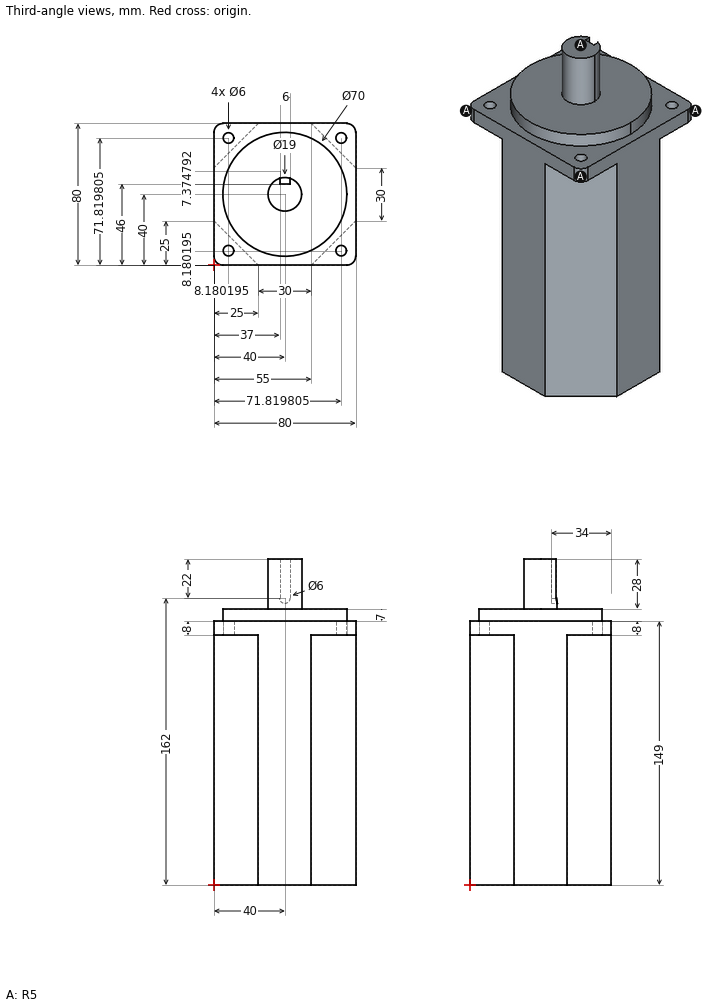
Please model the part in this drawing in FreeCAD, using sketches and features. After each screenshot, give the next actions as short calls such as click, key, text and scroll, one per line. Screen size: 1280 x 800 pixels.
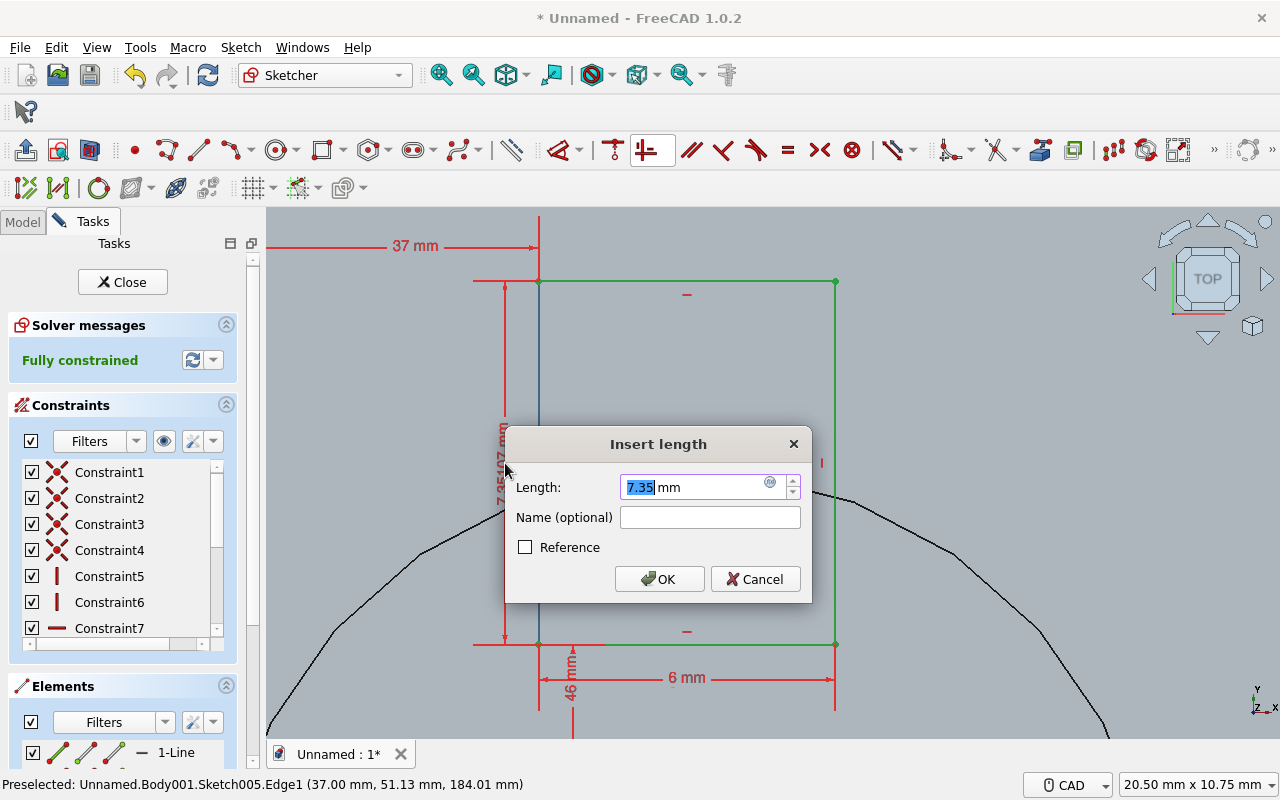
text(7.374792)
key(Return)
key(Escape)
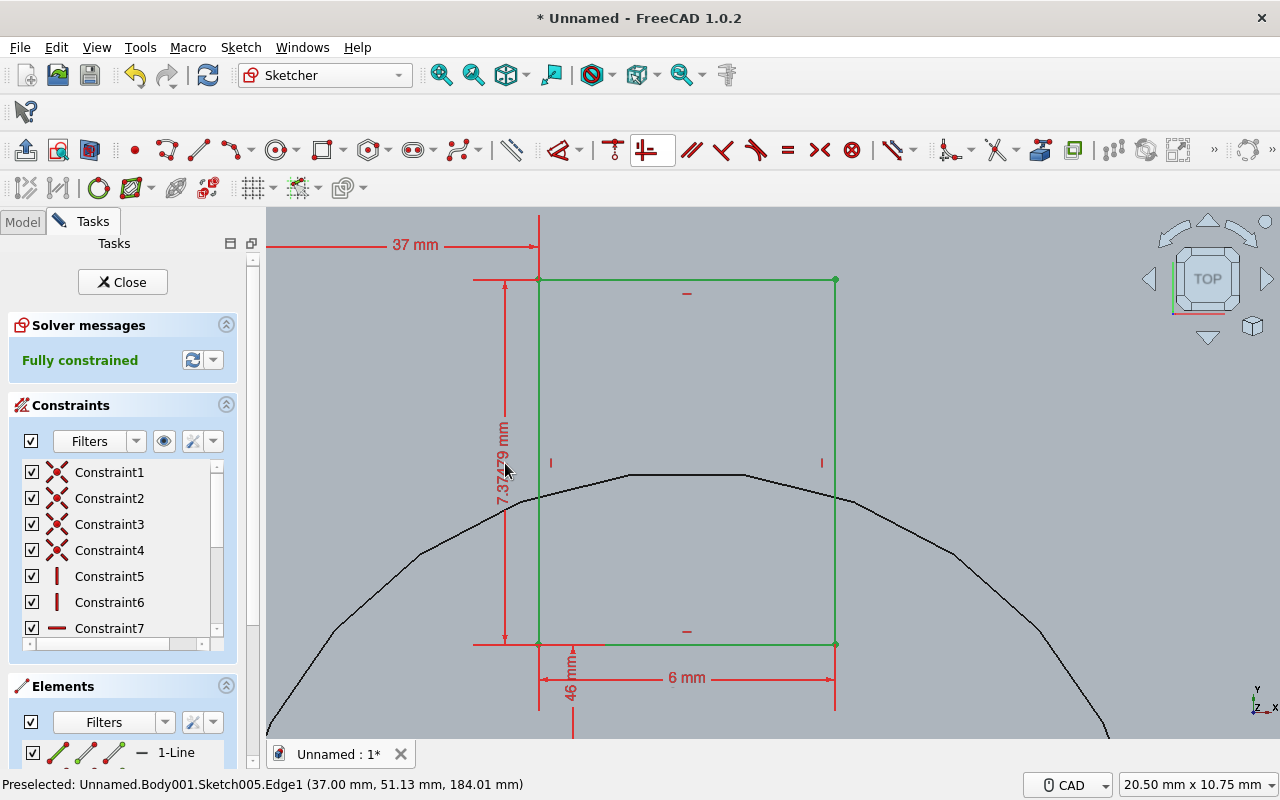
click(123, 282)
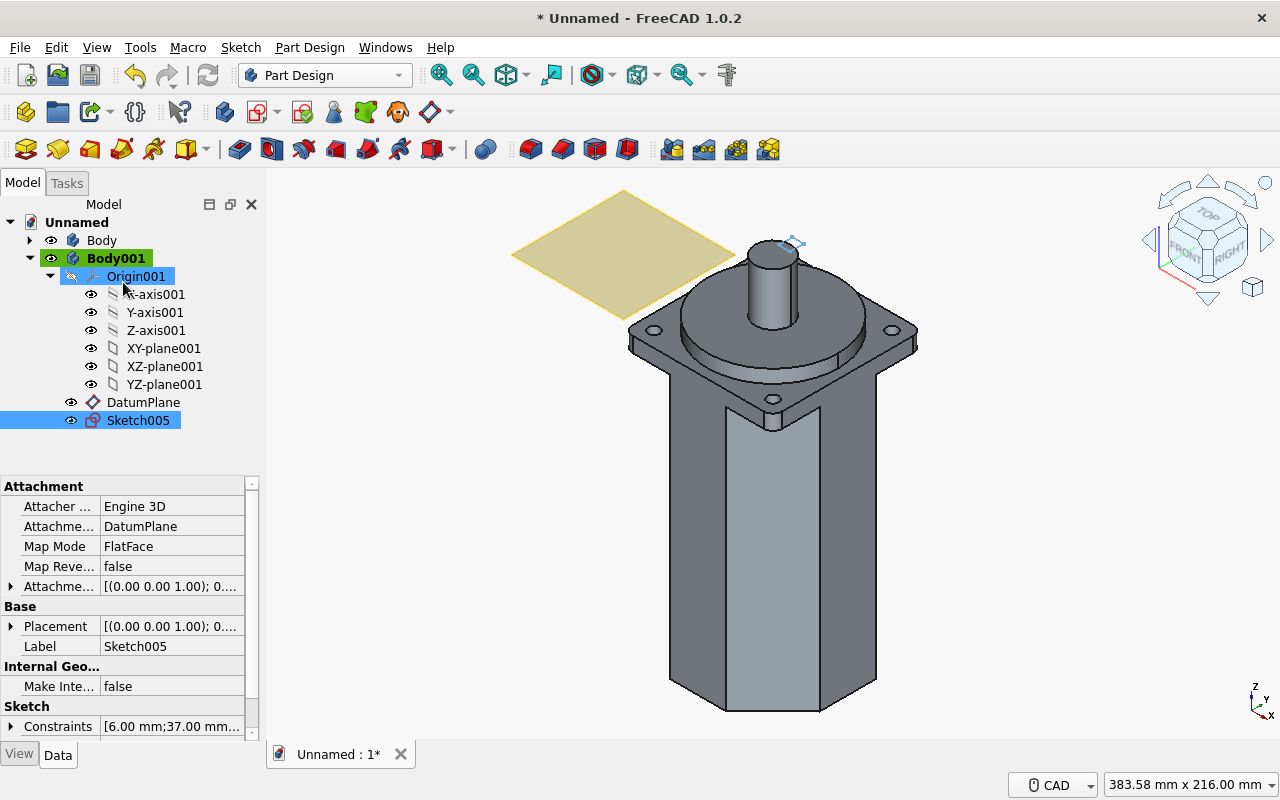
click(26, 150)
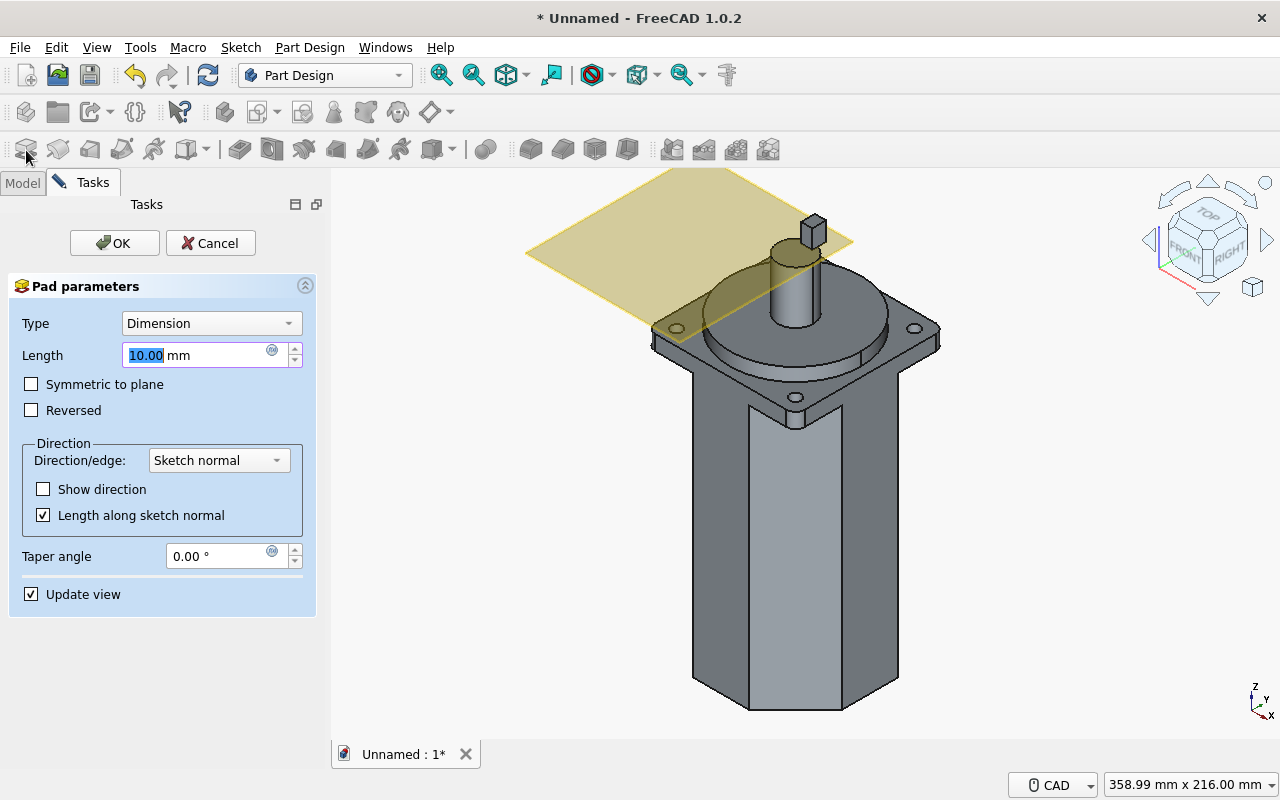
text(22)
key(Tab)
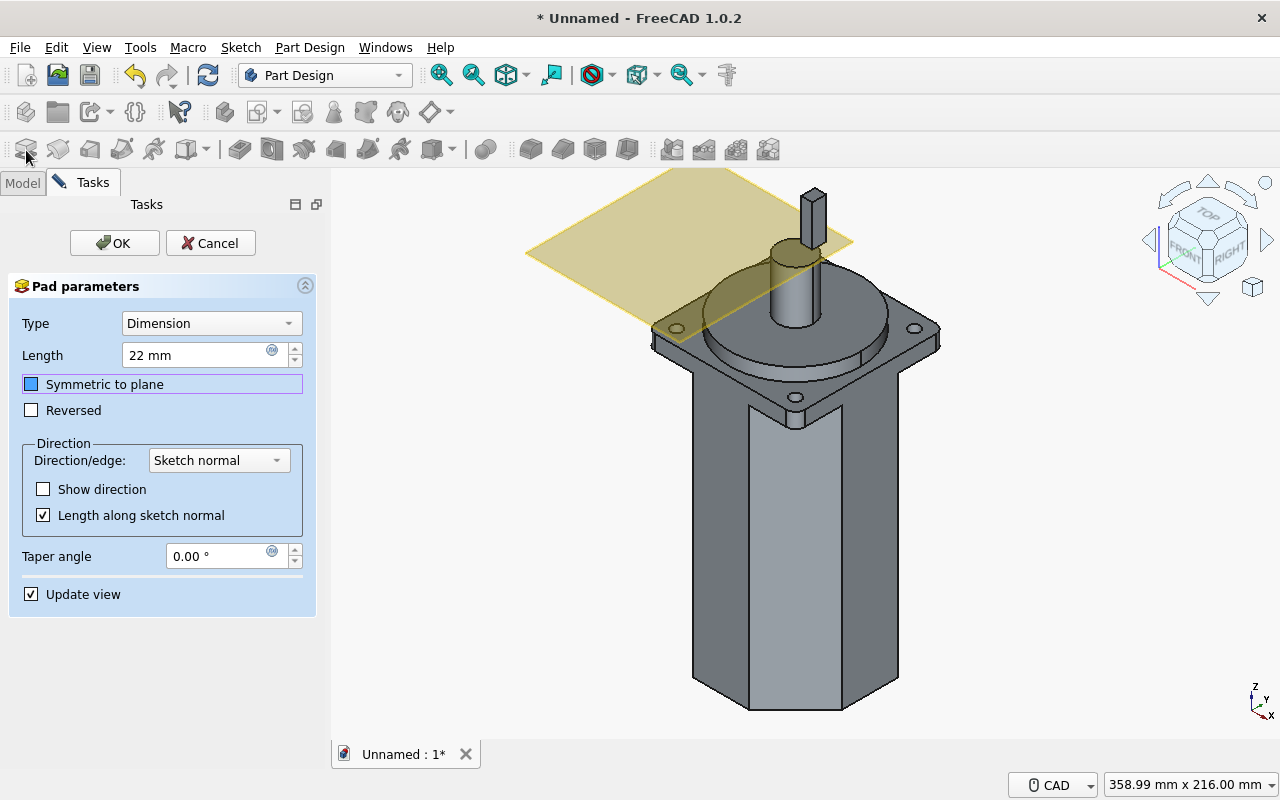
click(30, 410)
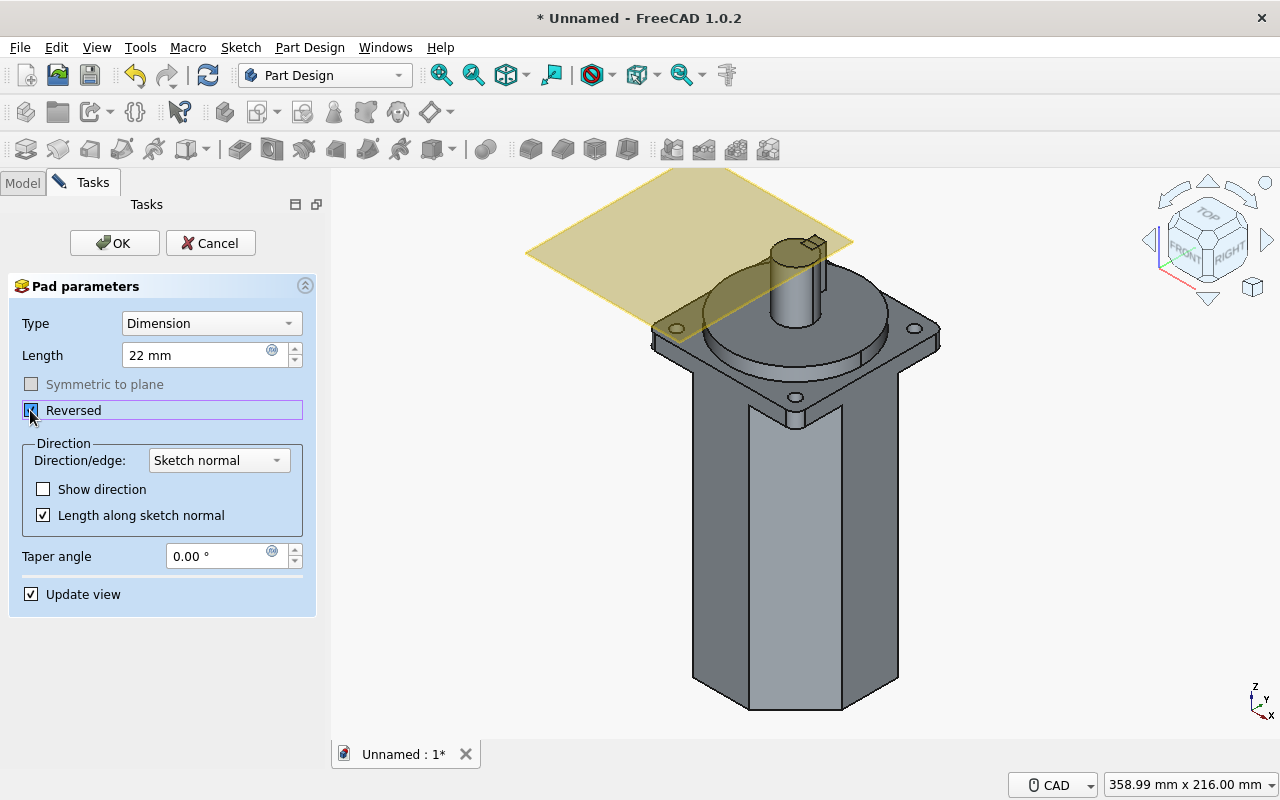
click(115, 243)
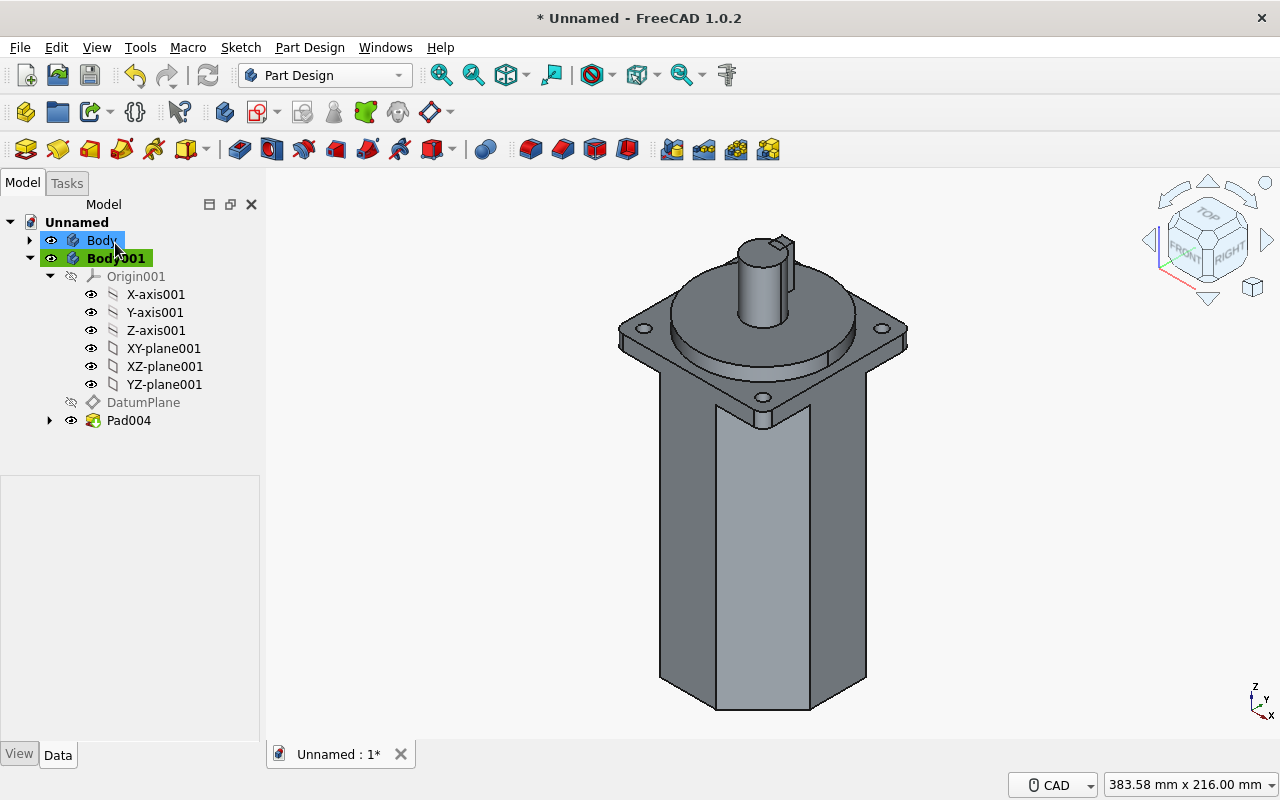
key(v)
key(f)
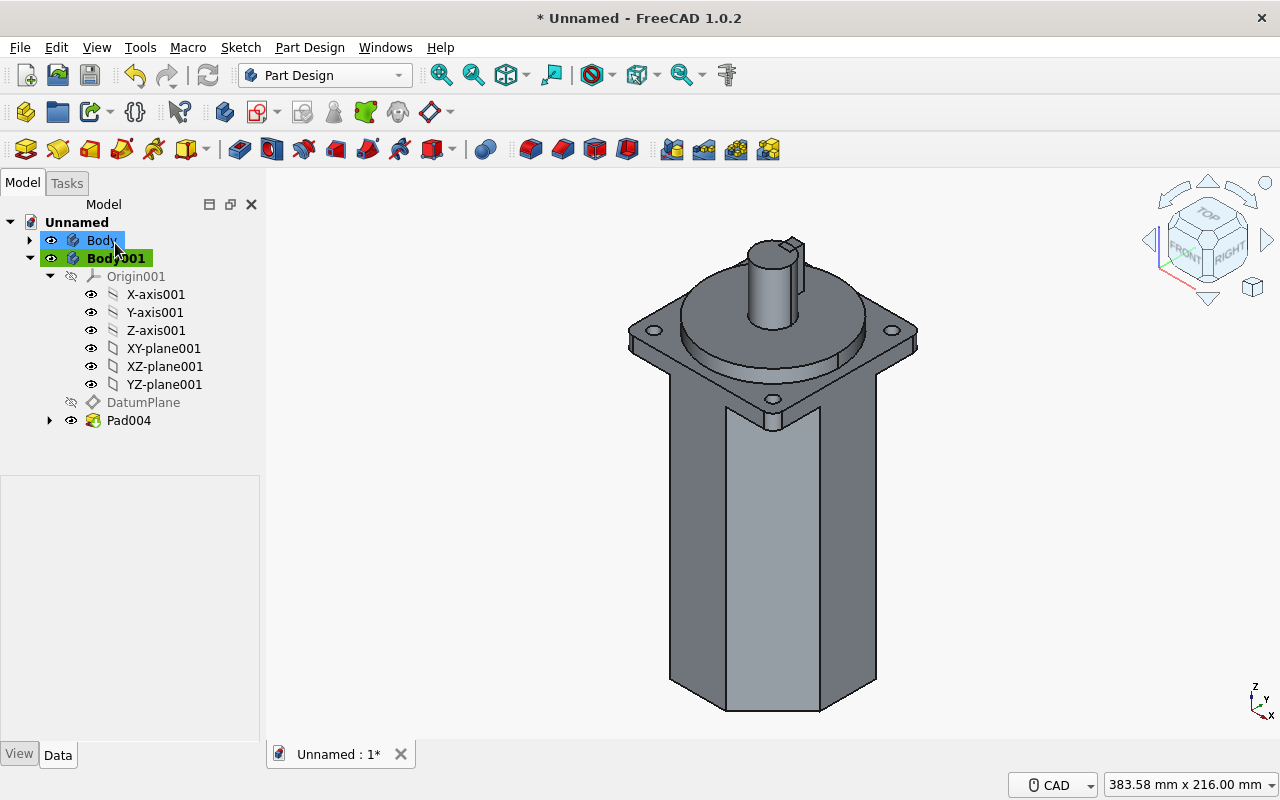
double_click(96, 240)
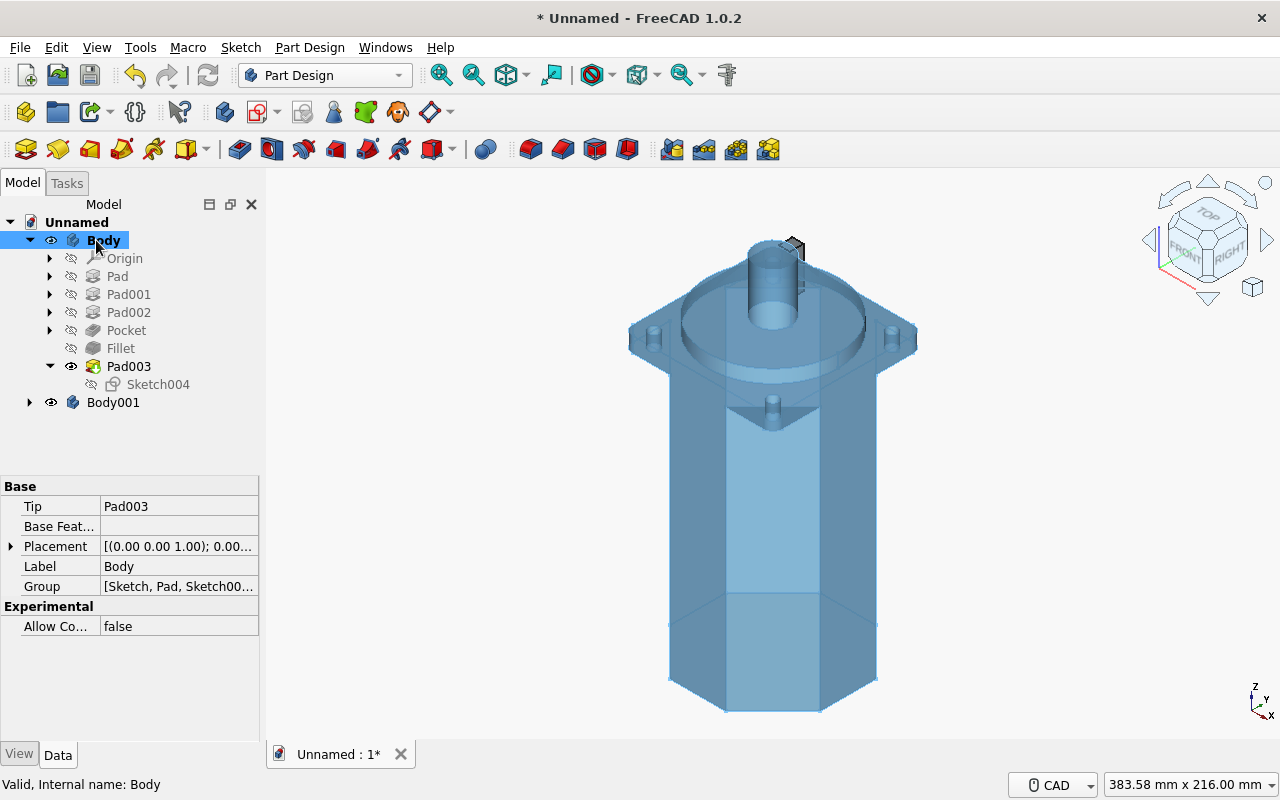
click(96, 402)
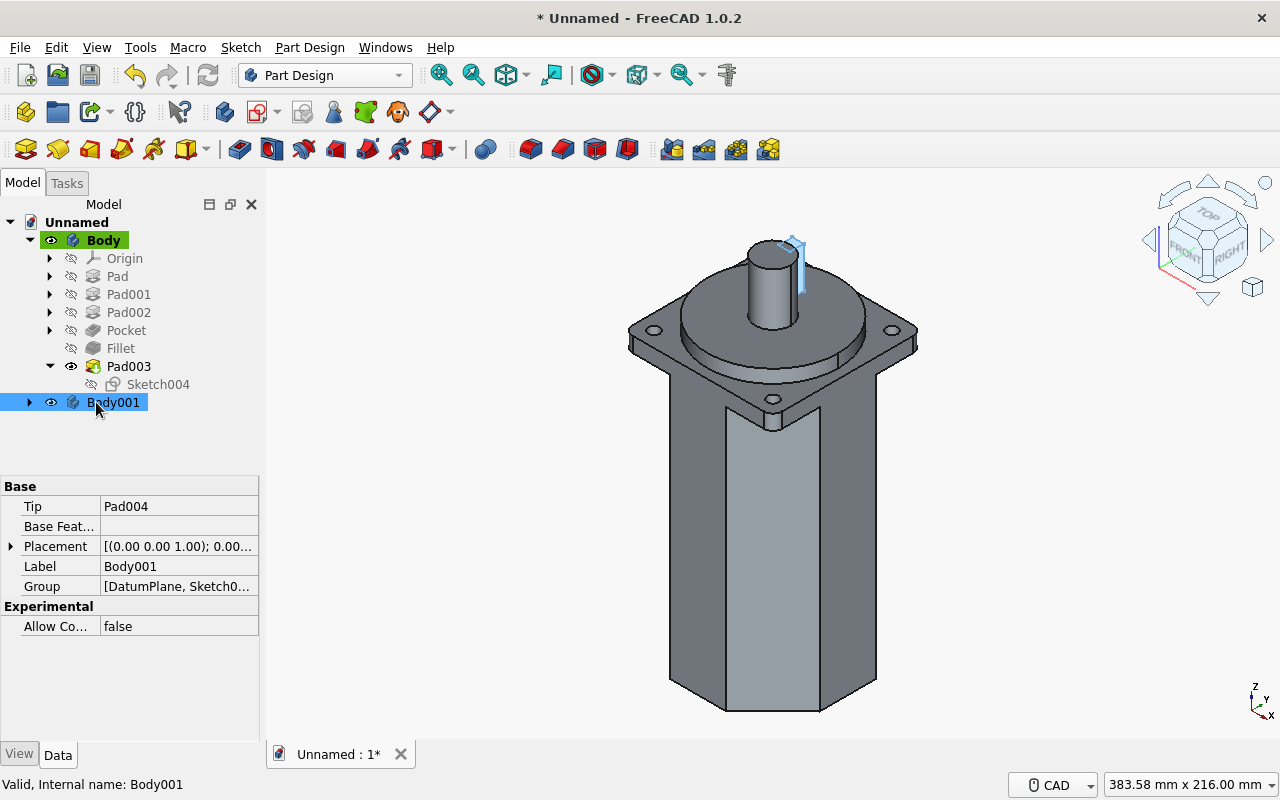
click(486, 150)